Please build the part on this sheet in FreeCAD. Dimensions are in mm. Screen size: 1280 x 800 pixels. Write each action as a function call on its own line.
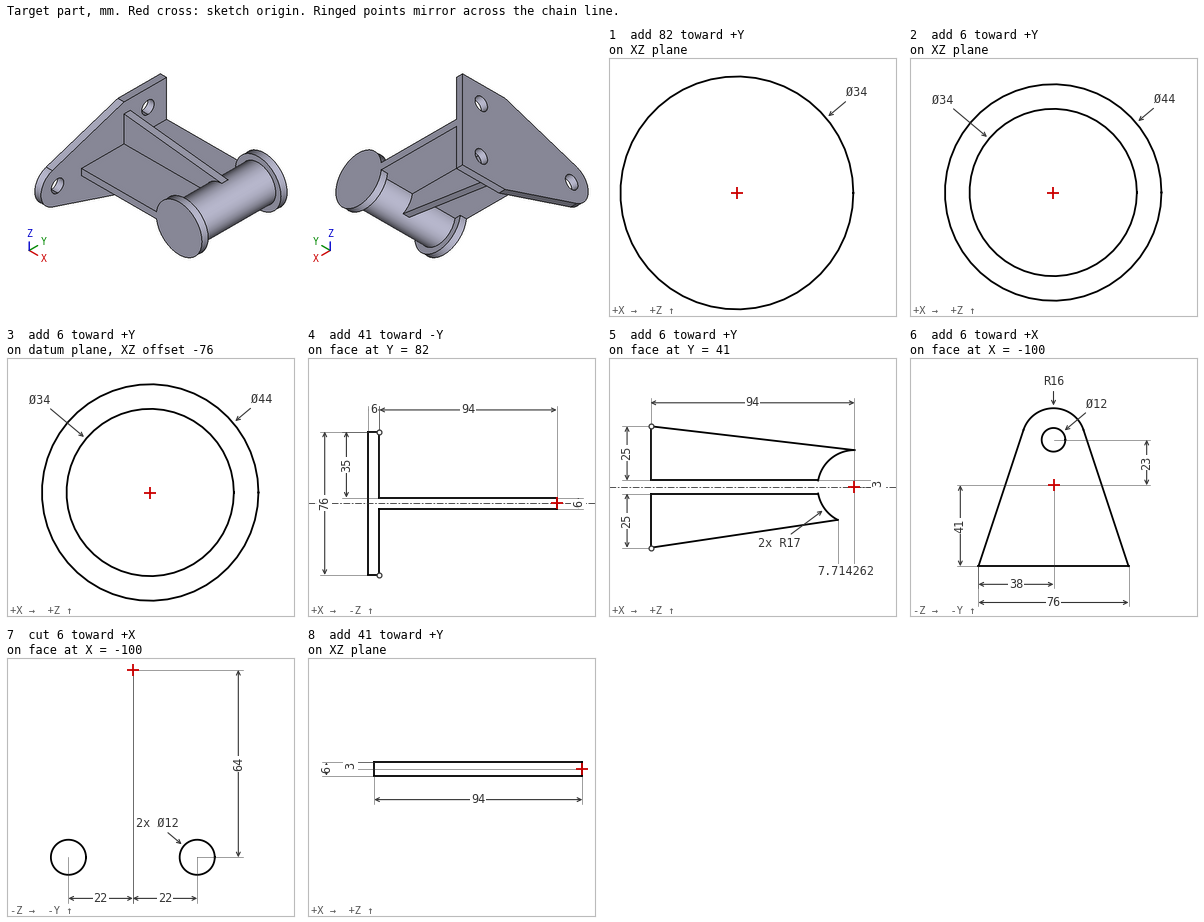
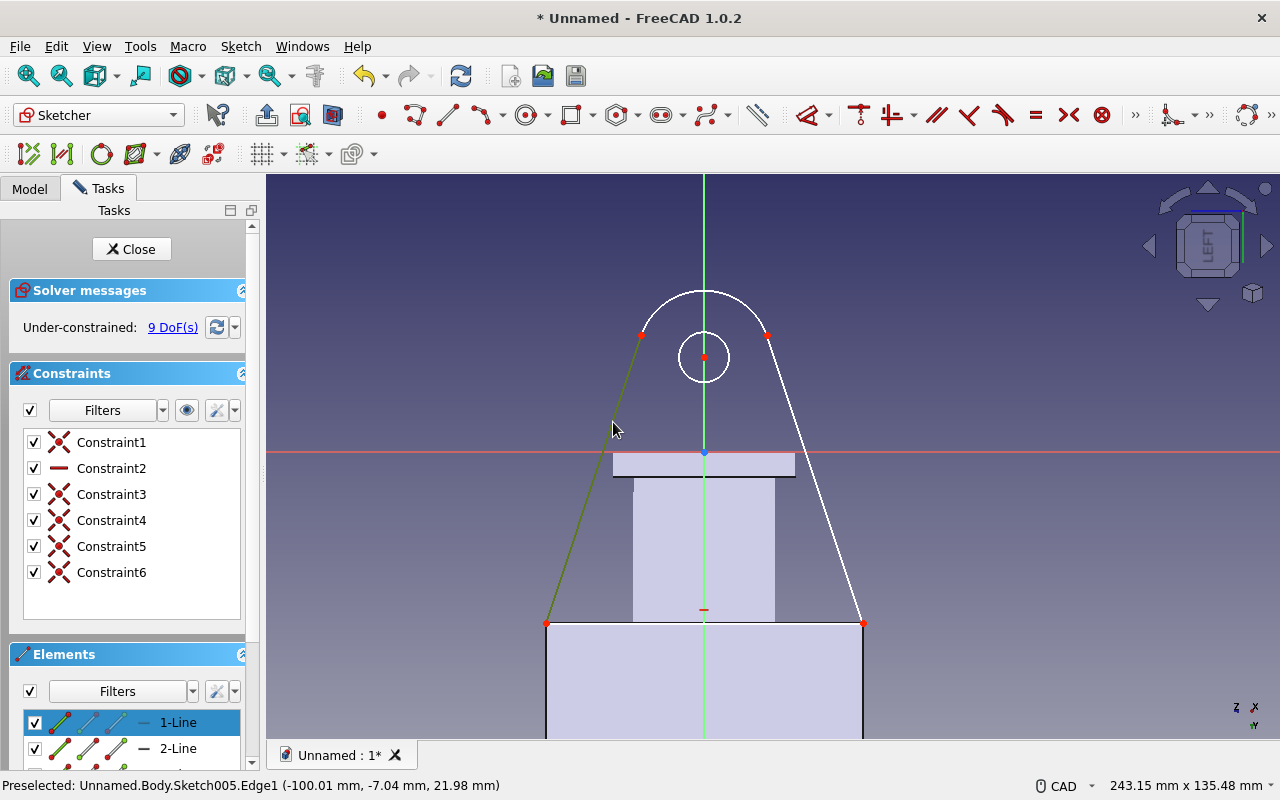
click(736, 299)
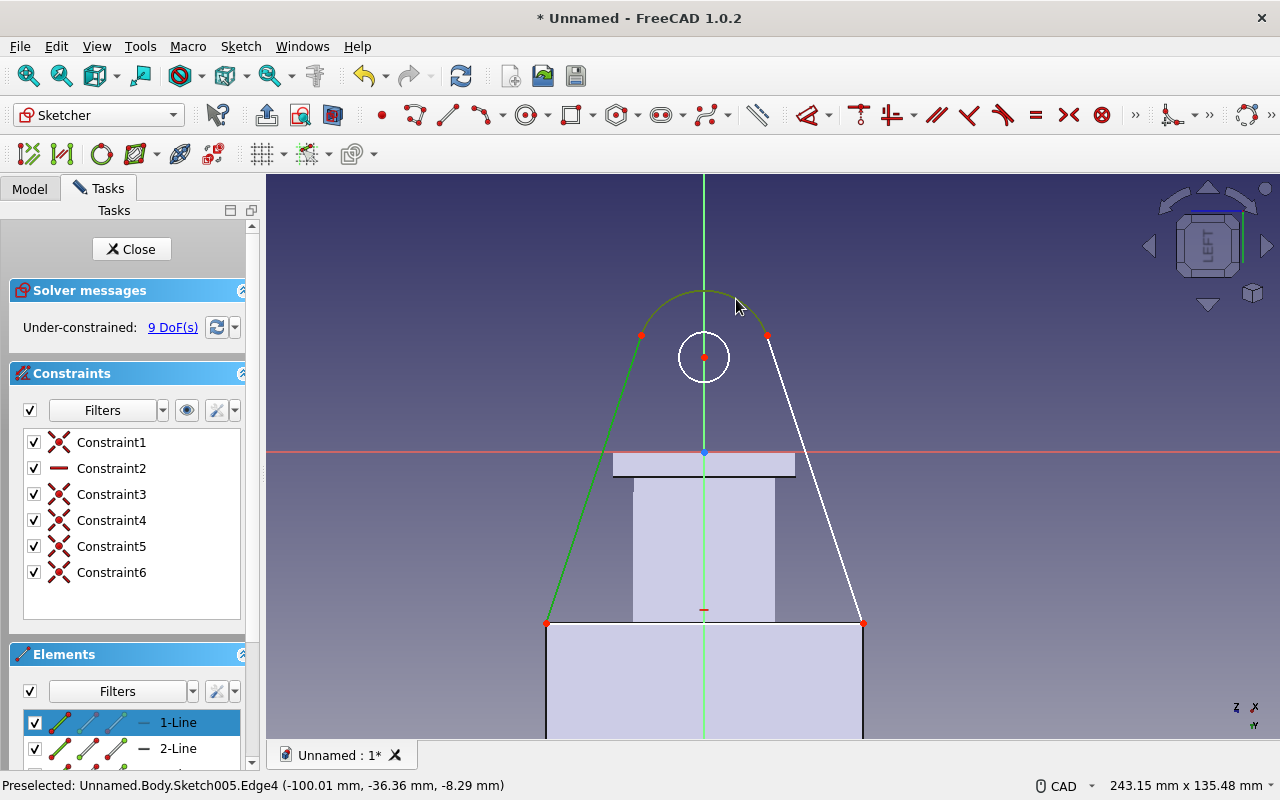
click(1003, 116)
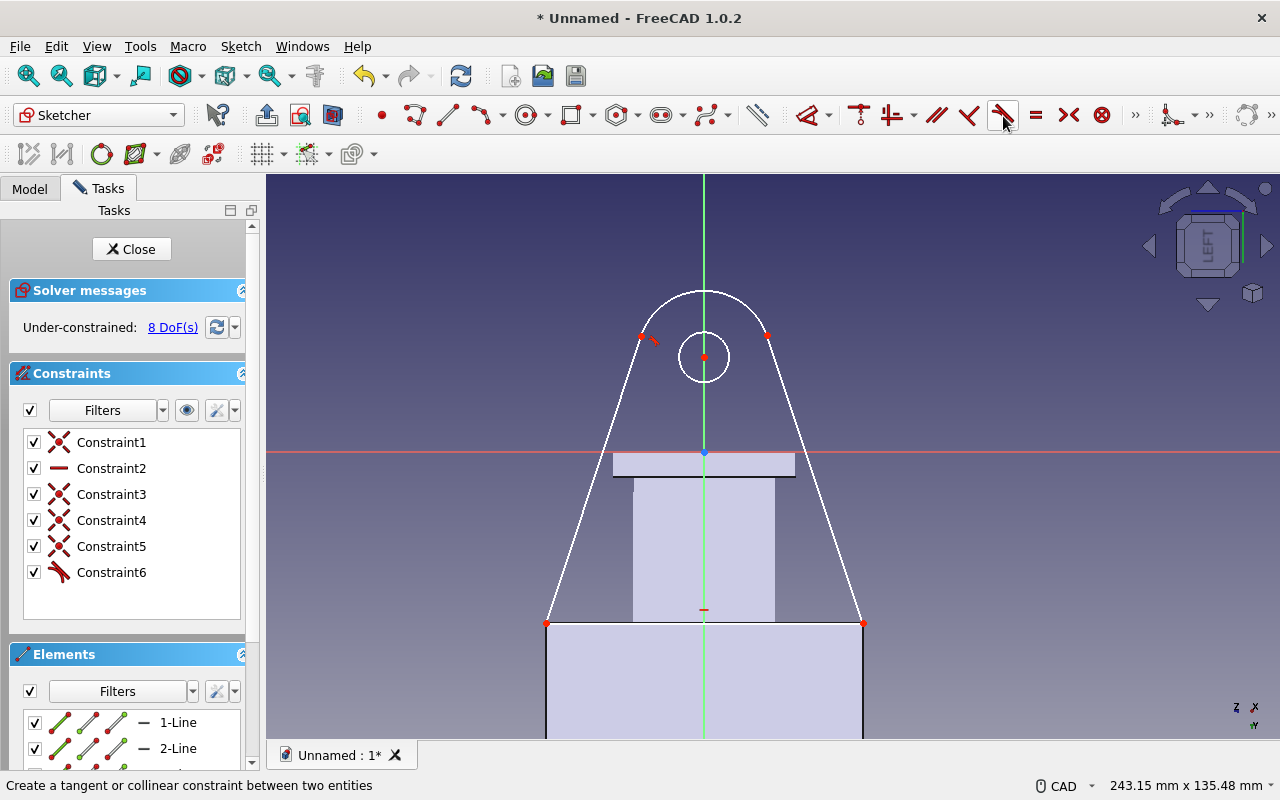
click(834, 538)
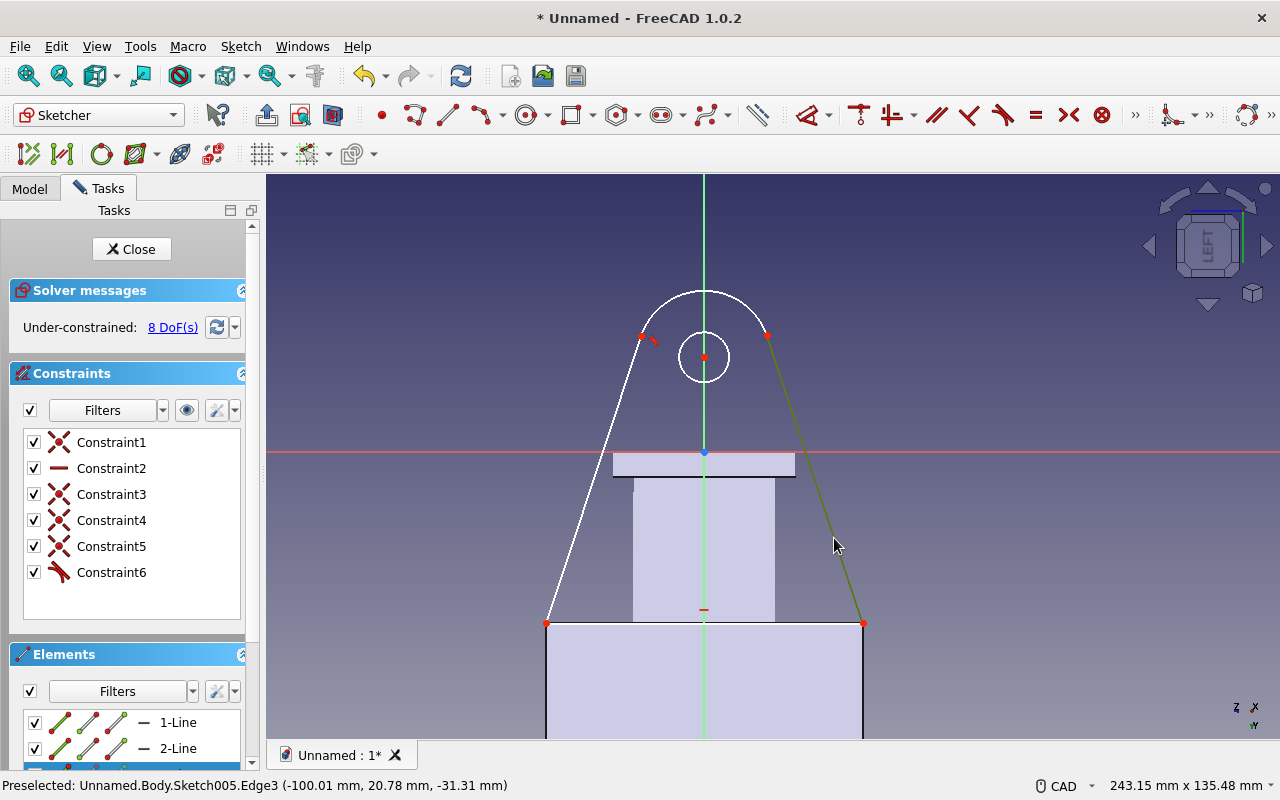
click(736, 299)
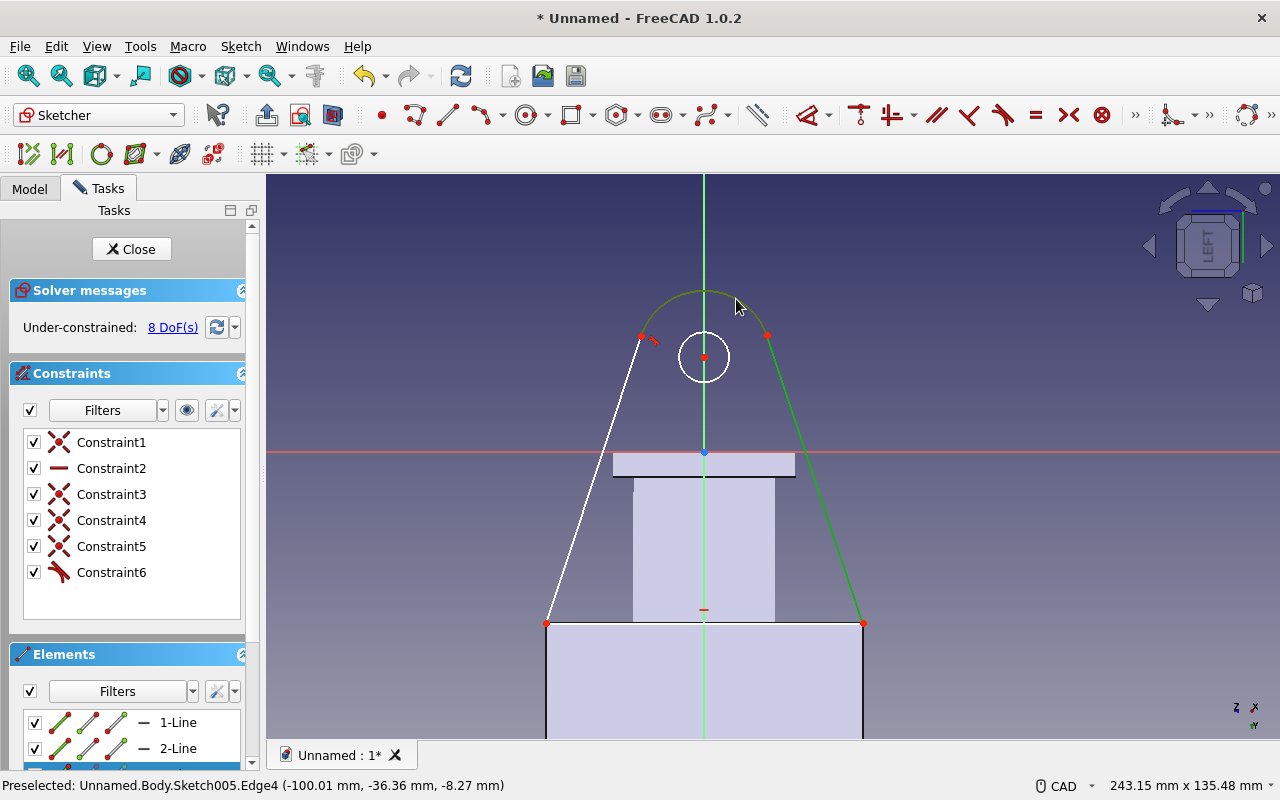
key(t)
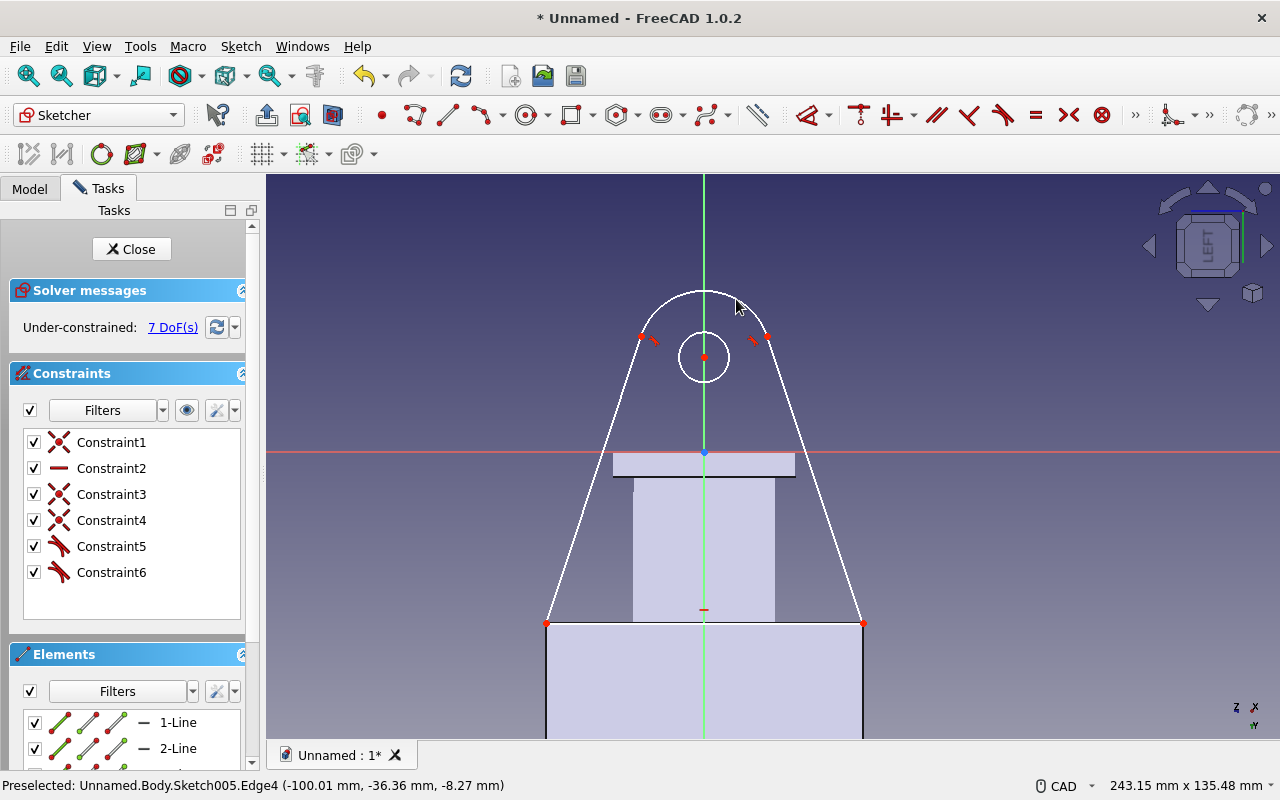
click(704, 357)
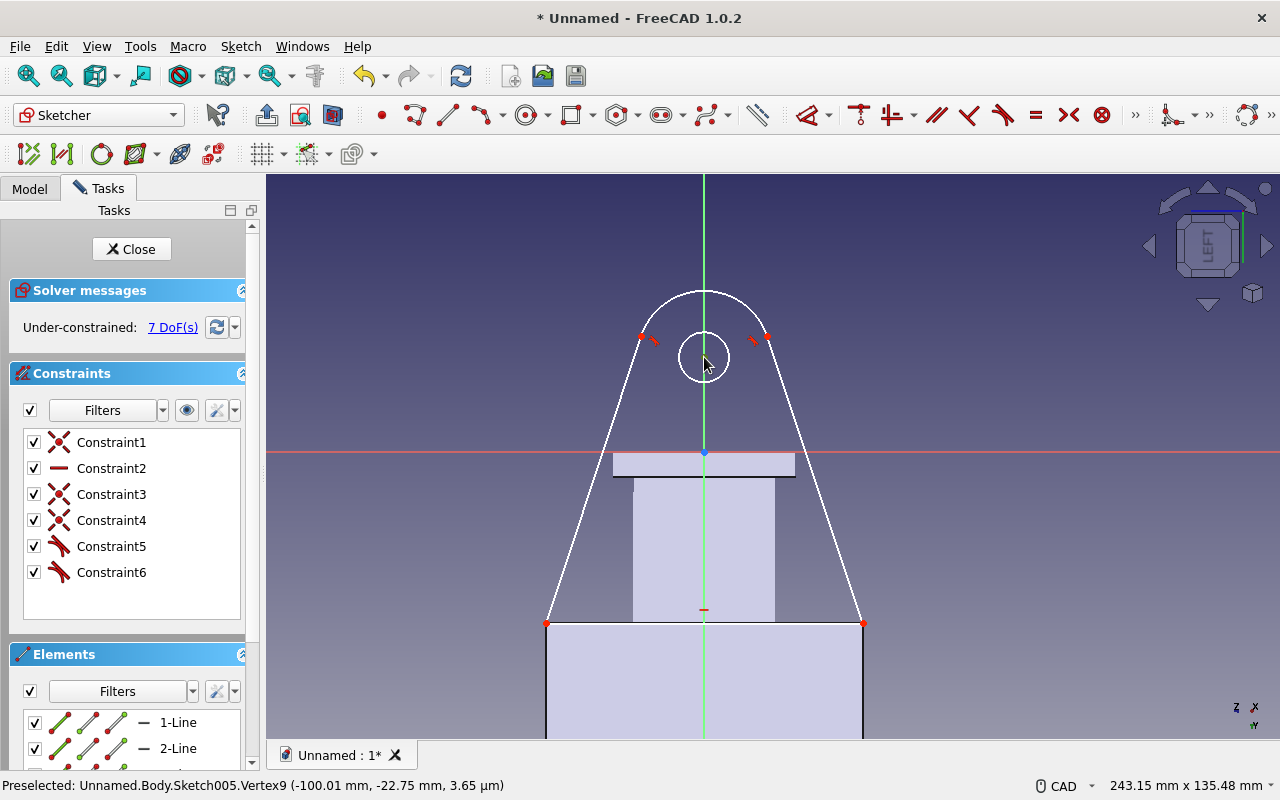
click(704, 675)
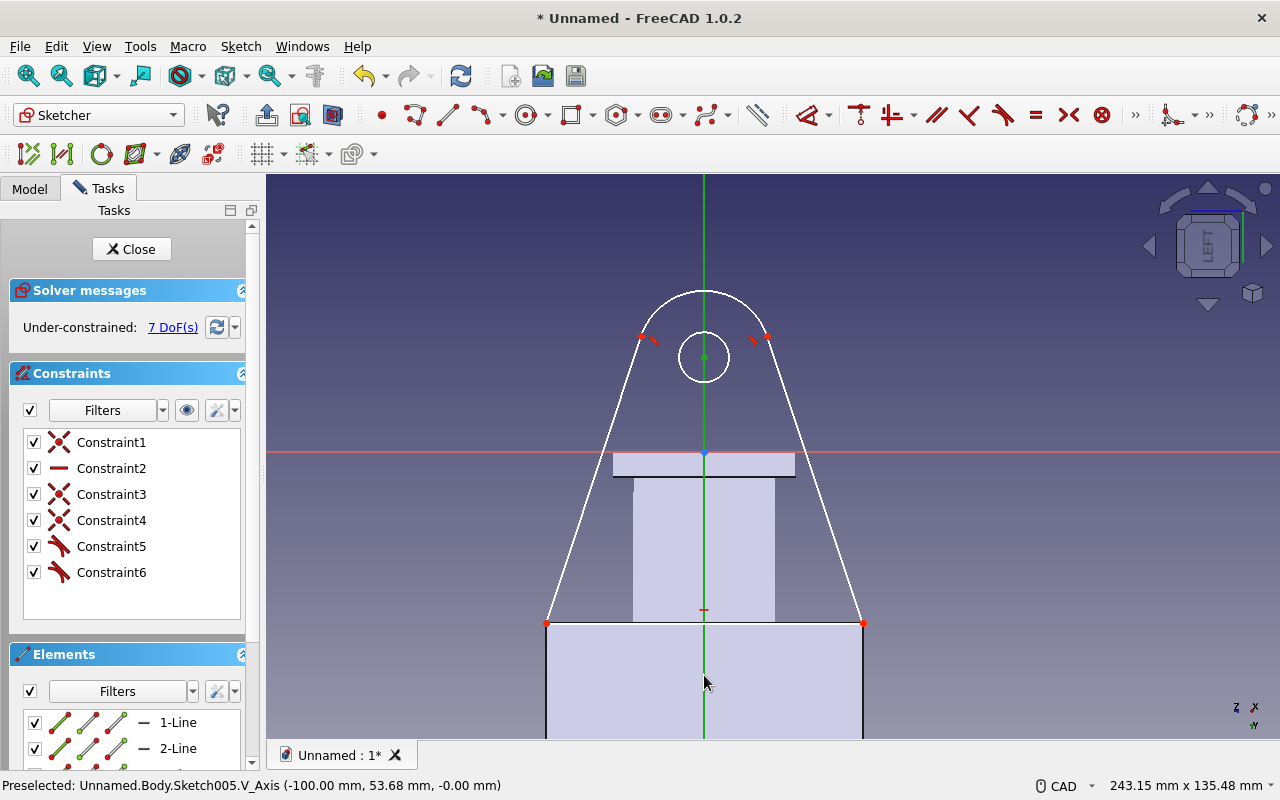
click(859, 116)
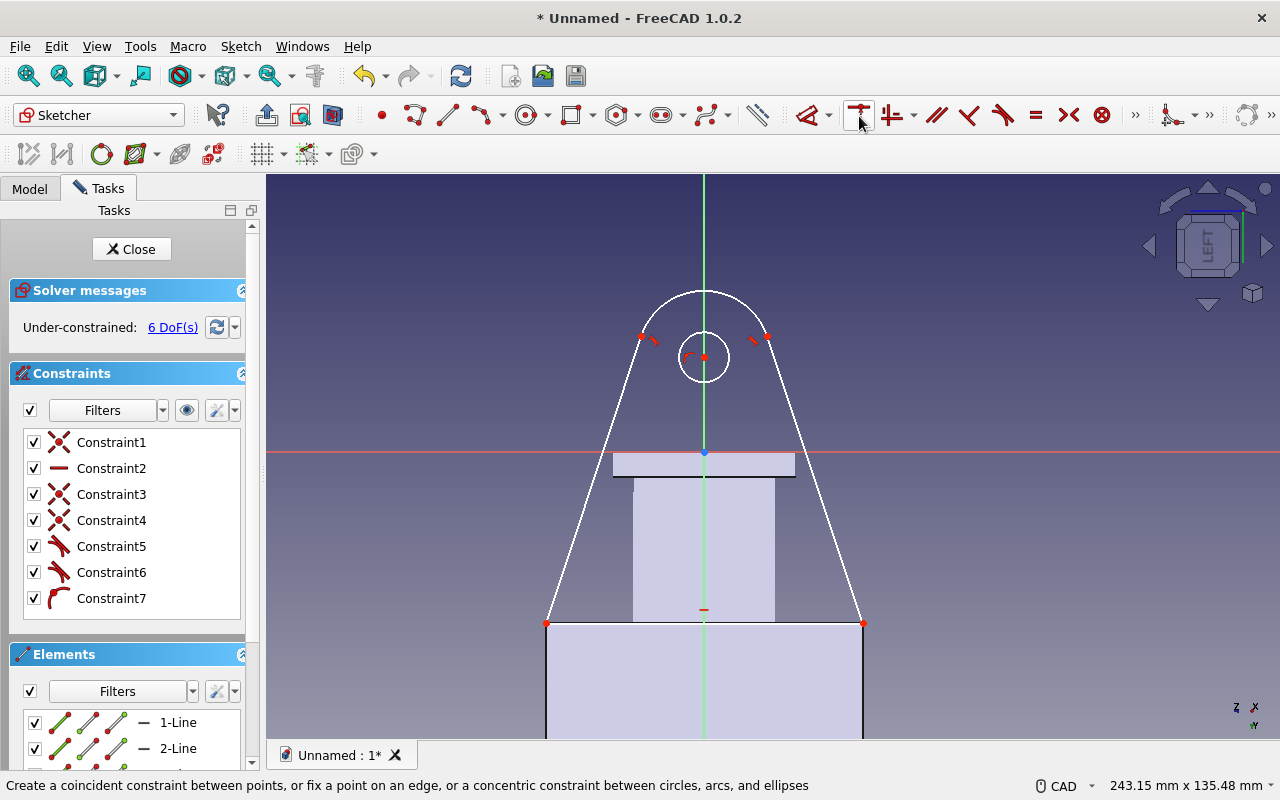
click(806, 116)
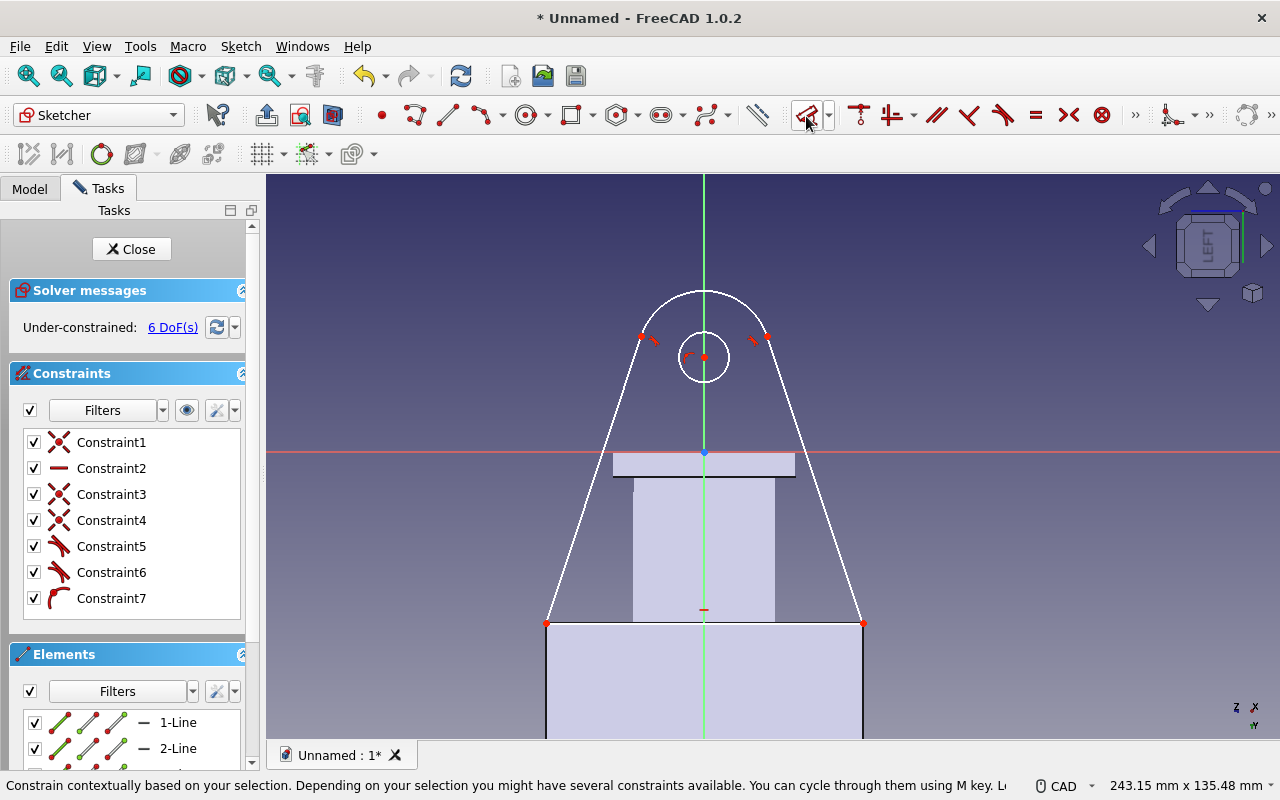
click(736, 299)
click(751, 271)